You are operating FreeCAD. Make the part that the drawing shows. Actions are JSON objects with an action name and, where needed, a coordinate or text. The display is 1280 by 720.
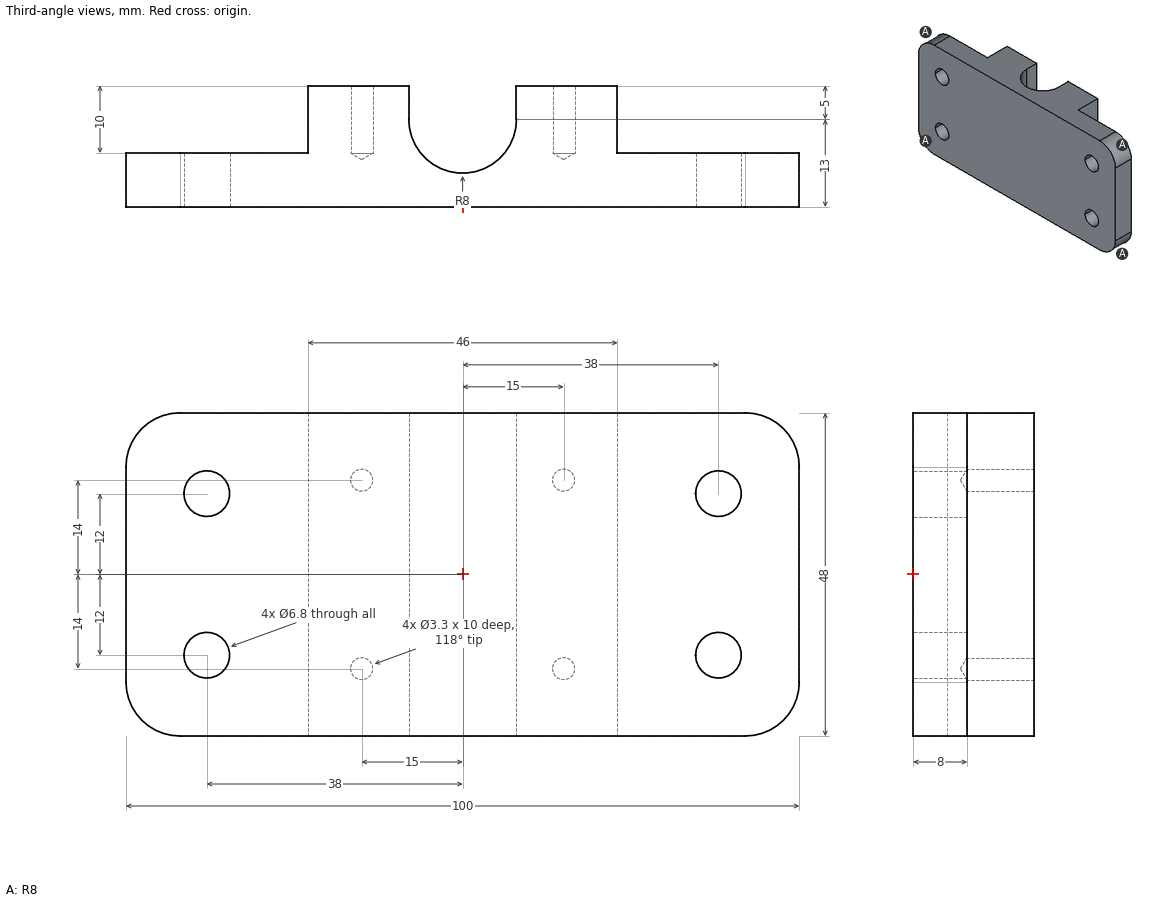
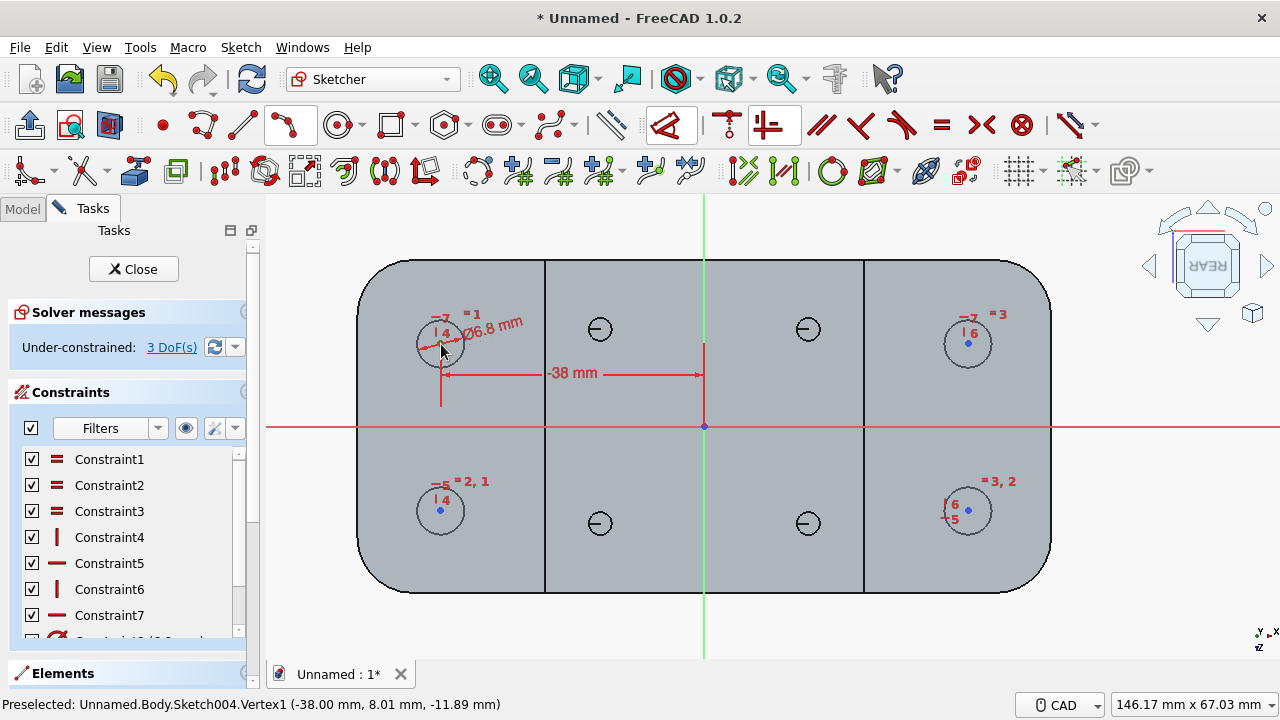
{"action": "left_click", "coordinate": [692, 126]}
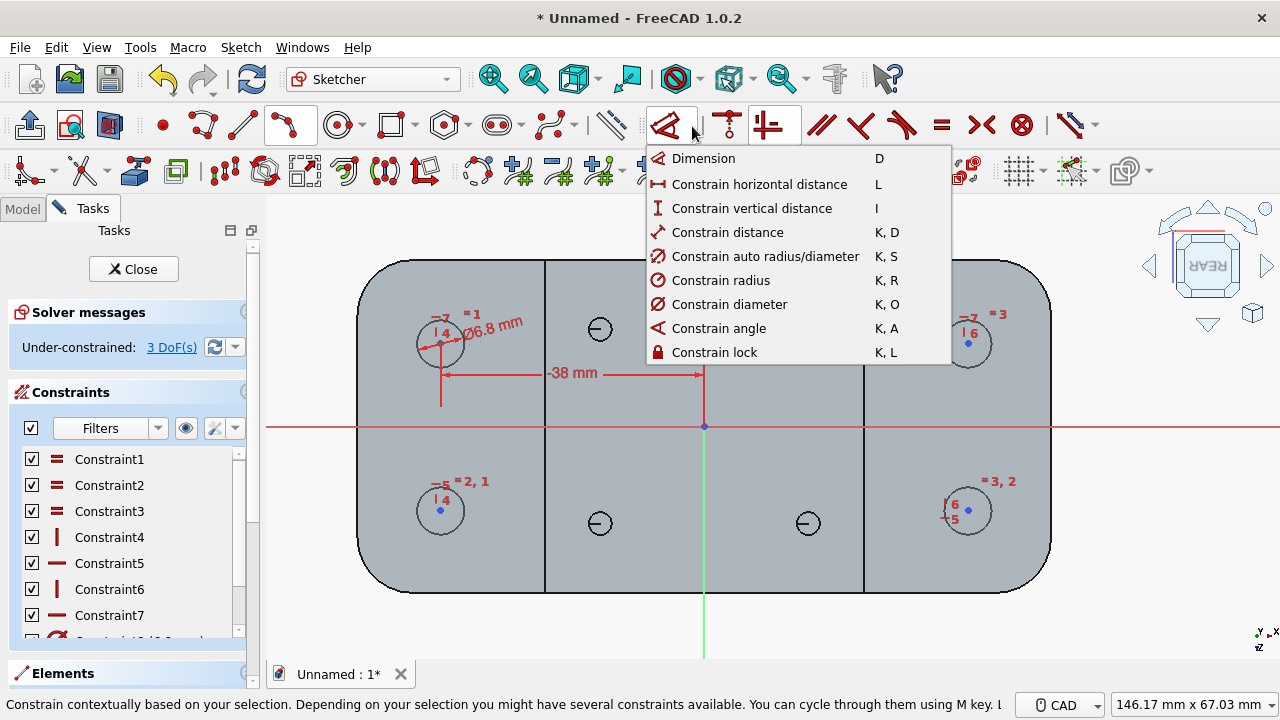
{"action": "left_click", "coordinate": [799, 208]}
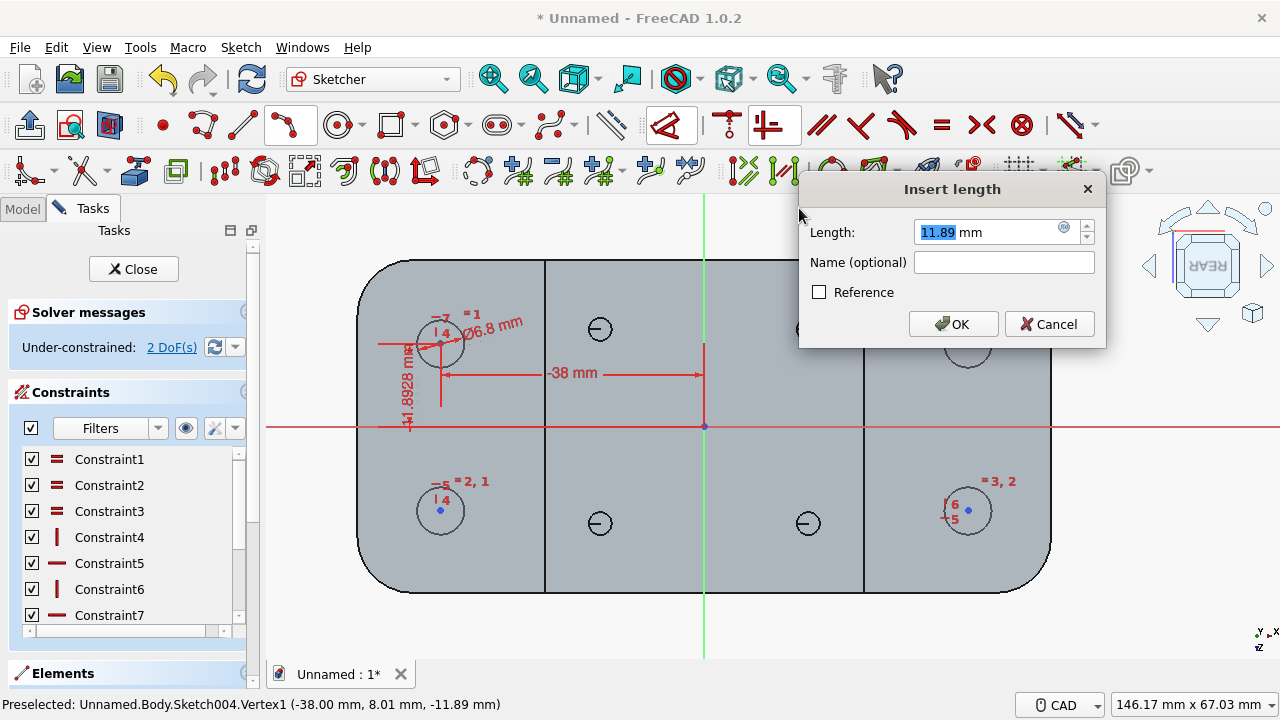
{"action": "type", "text": "12"}
{"action": "key", "text": "Return"}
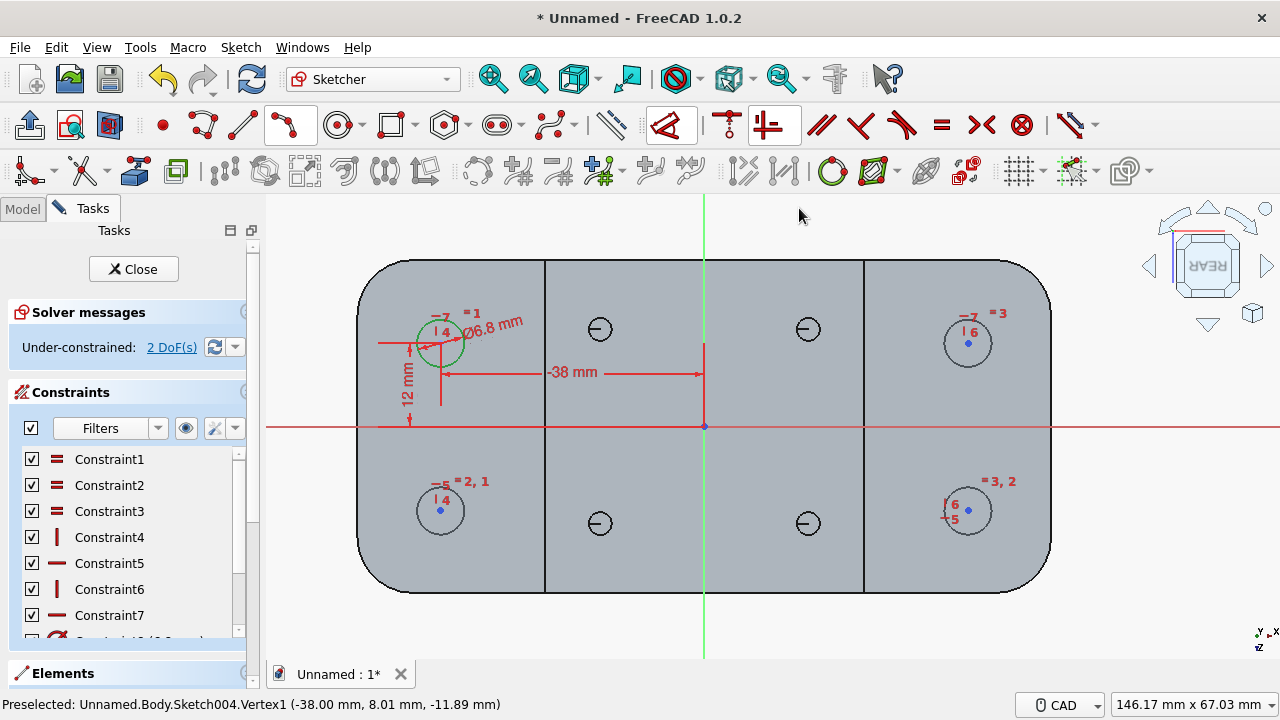
{"action": "left_click", "coordinate": [441, 511]}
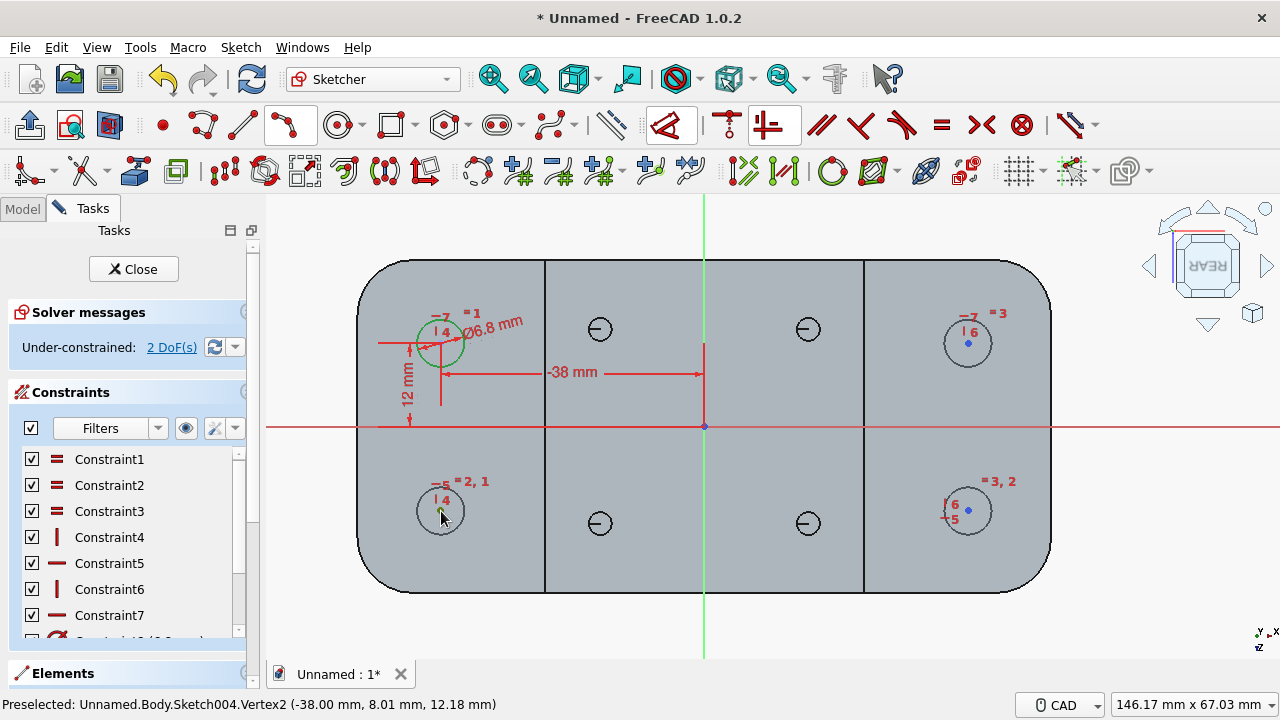
{"action": "left_click", "coordinate": [692, 126]}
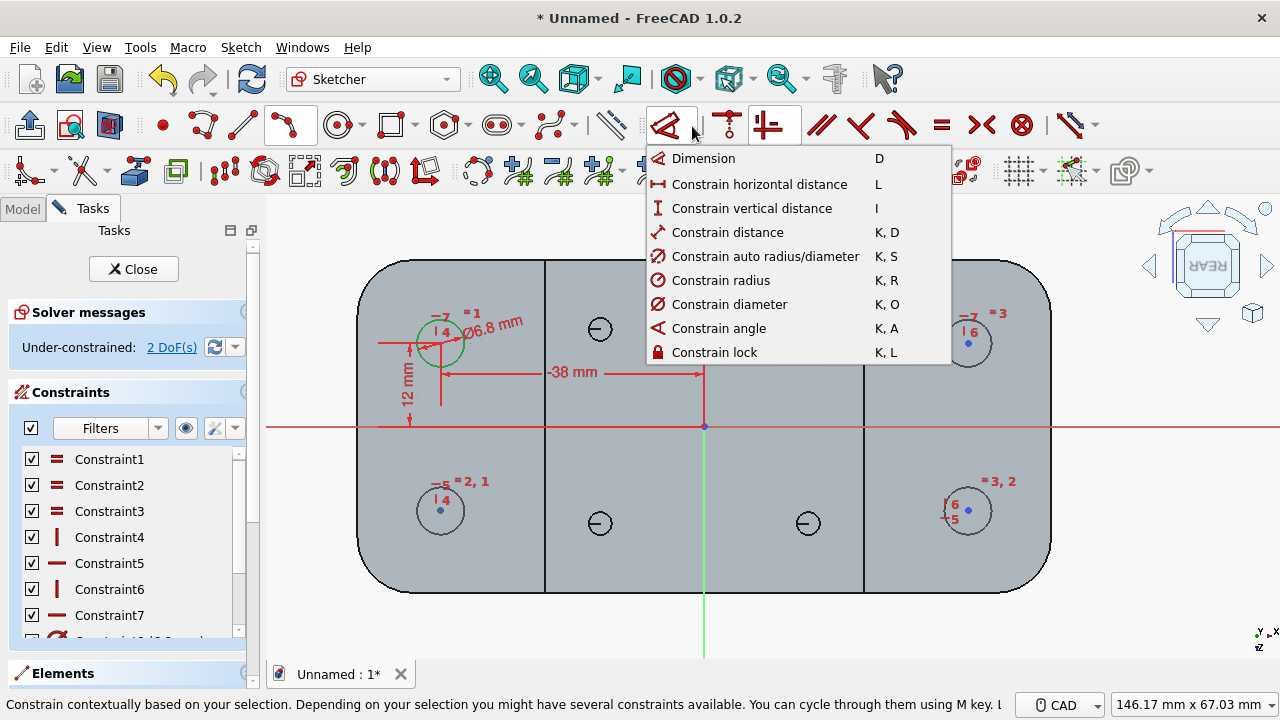
{"action": "left_click", "coordinate": [799, 208]}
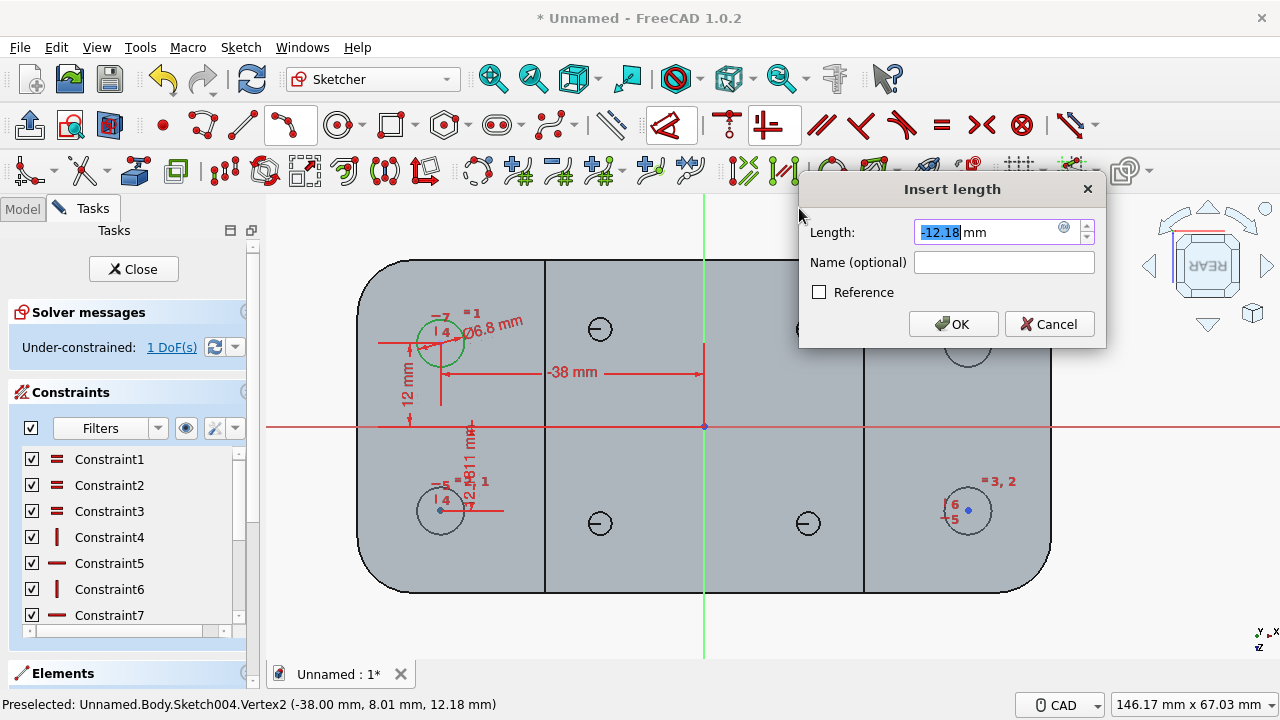
{"action": "type", "text": "-12"}
{"action": "key", "text": "Return"}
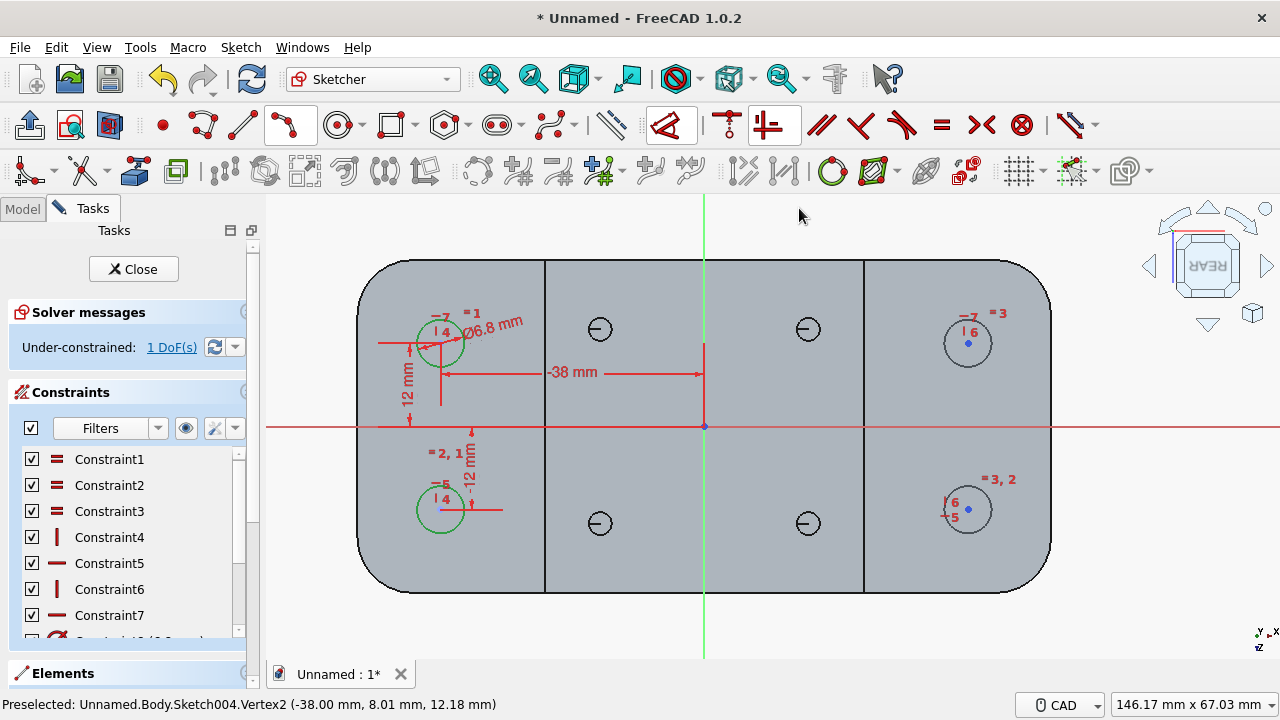
{"action": "left_click", "coordinate": [968, 510]}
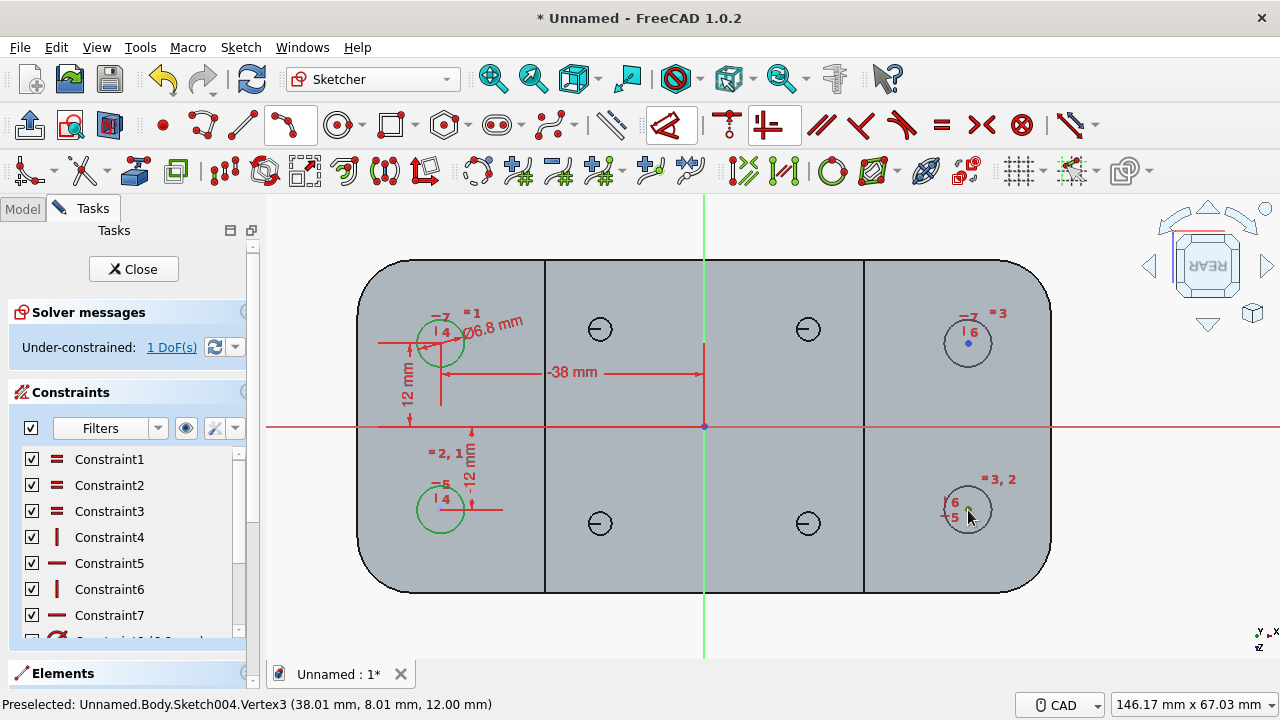
{"action": "key", "text": "l"}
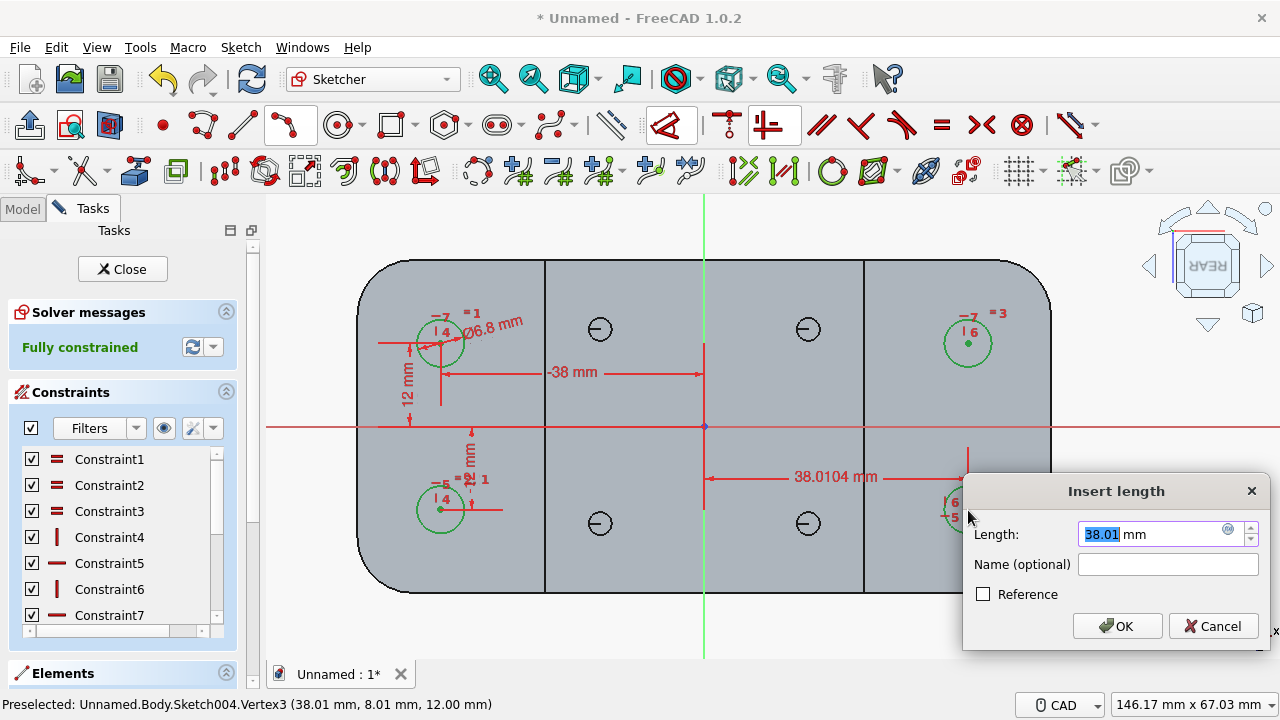
{"action": "type", "text": "38"}
{"action": "key", "text": "Return"}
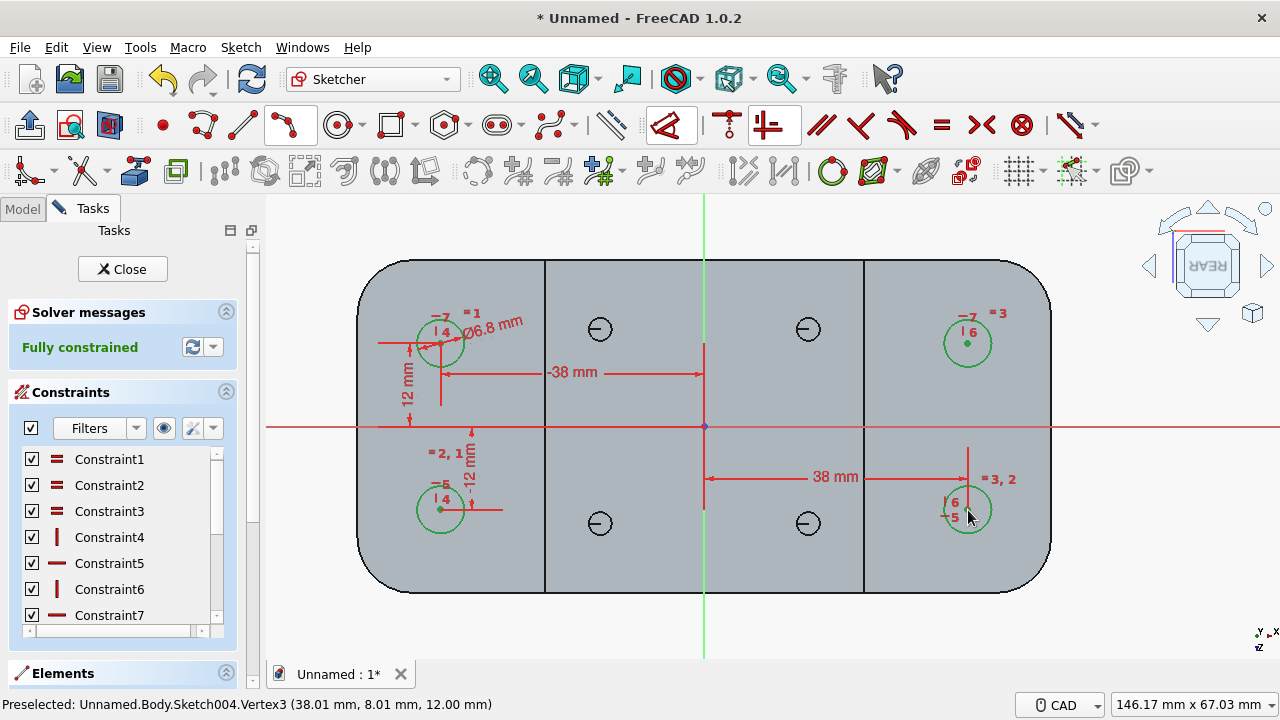
{"action": "left_click", "coordinate": [123, 269]}